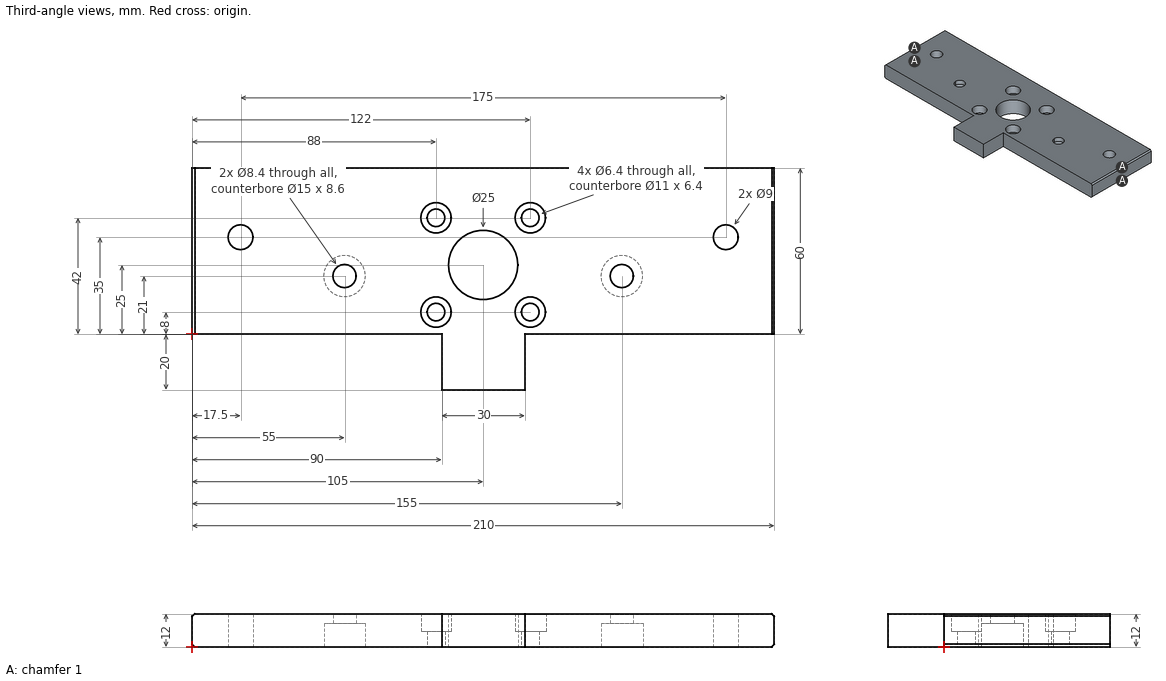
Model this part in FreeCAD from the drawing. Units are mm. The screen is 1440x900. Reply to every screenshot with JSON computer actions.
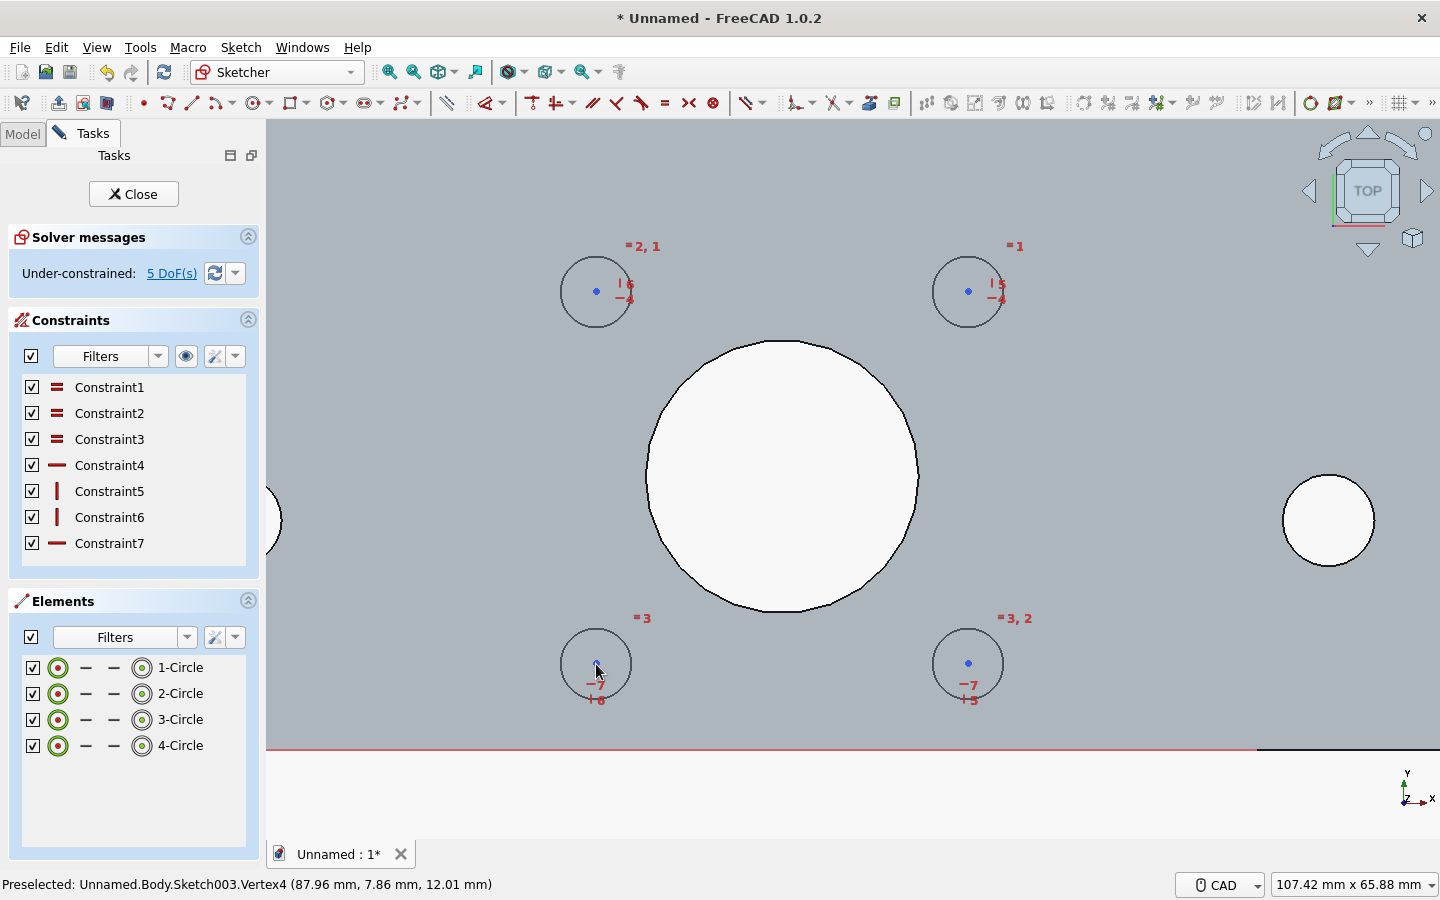
{"action": "key", "text": "d"}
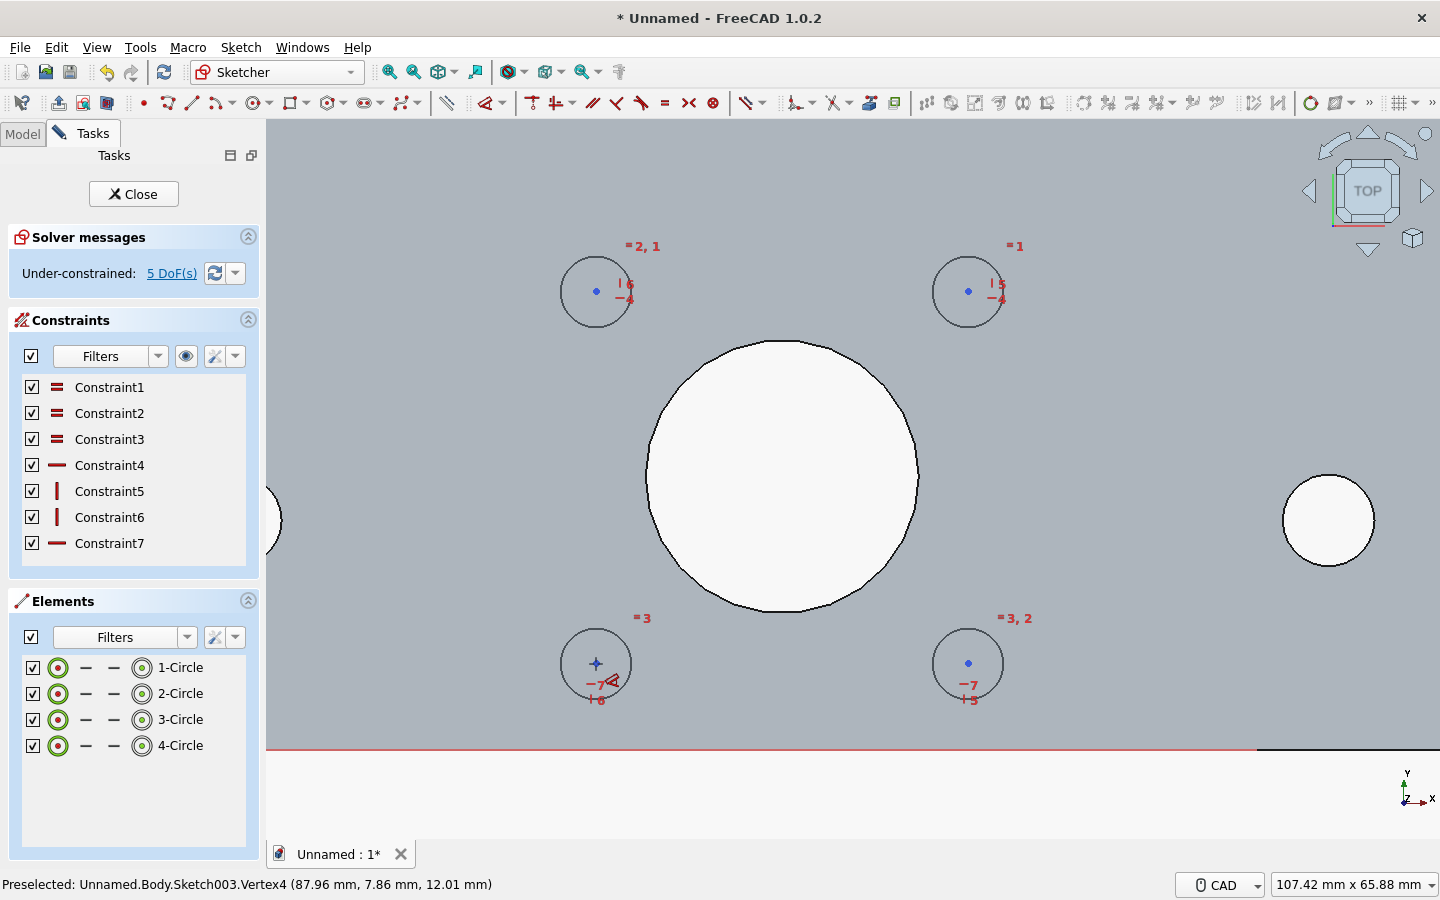
{"action": "left_click", "coordinate": [993, 267]}
{"action": "left_click", "coordinate": [1016, 244]}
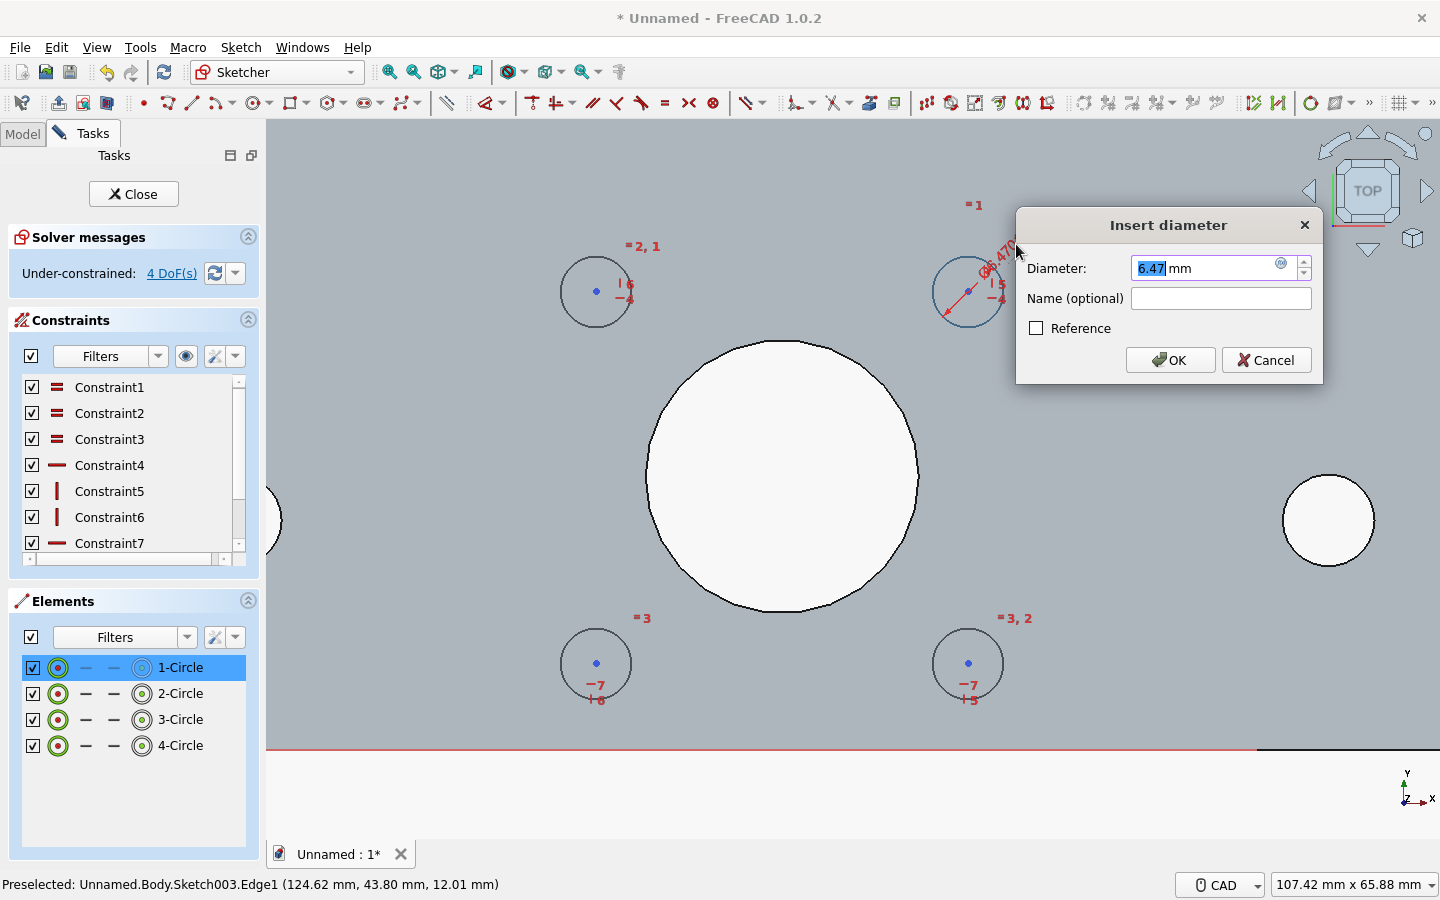
{"action": "type", "text": "6.4"}
{"action": "key", "text": "Return"}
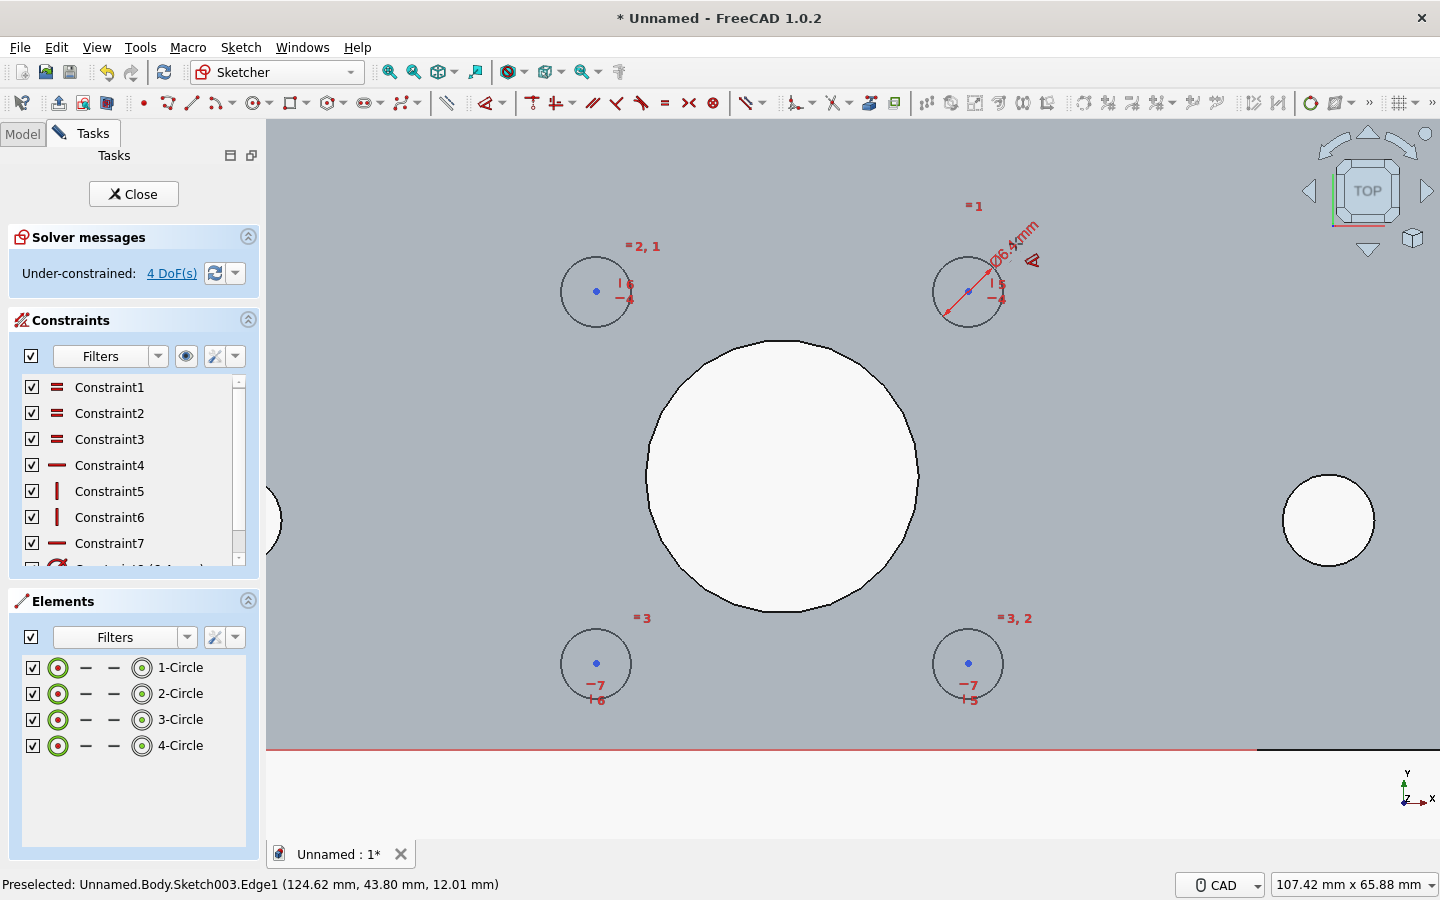
{"action": "left_click", "coordinate": [968, 664]}
{"action": "left_click", "coordinate": [1002, 707]}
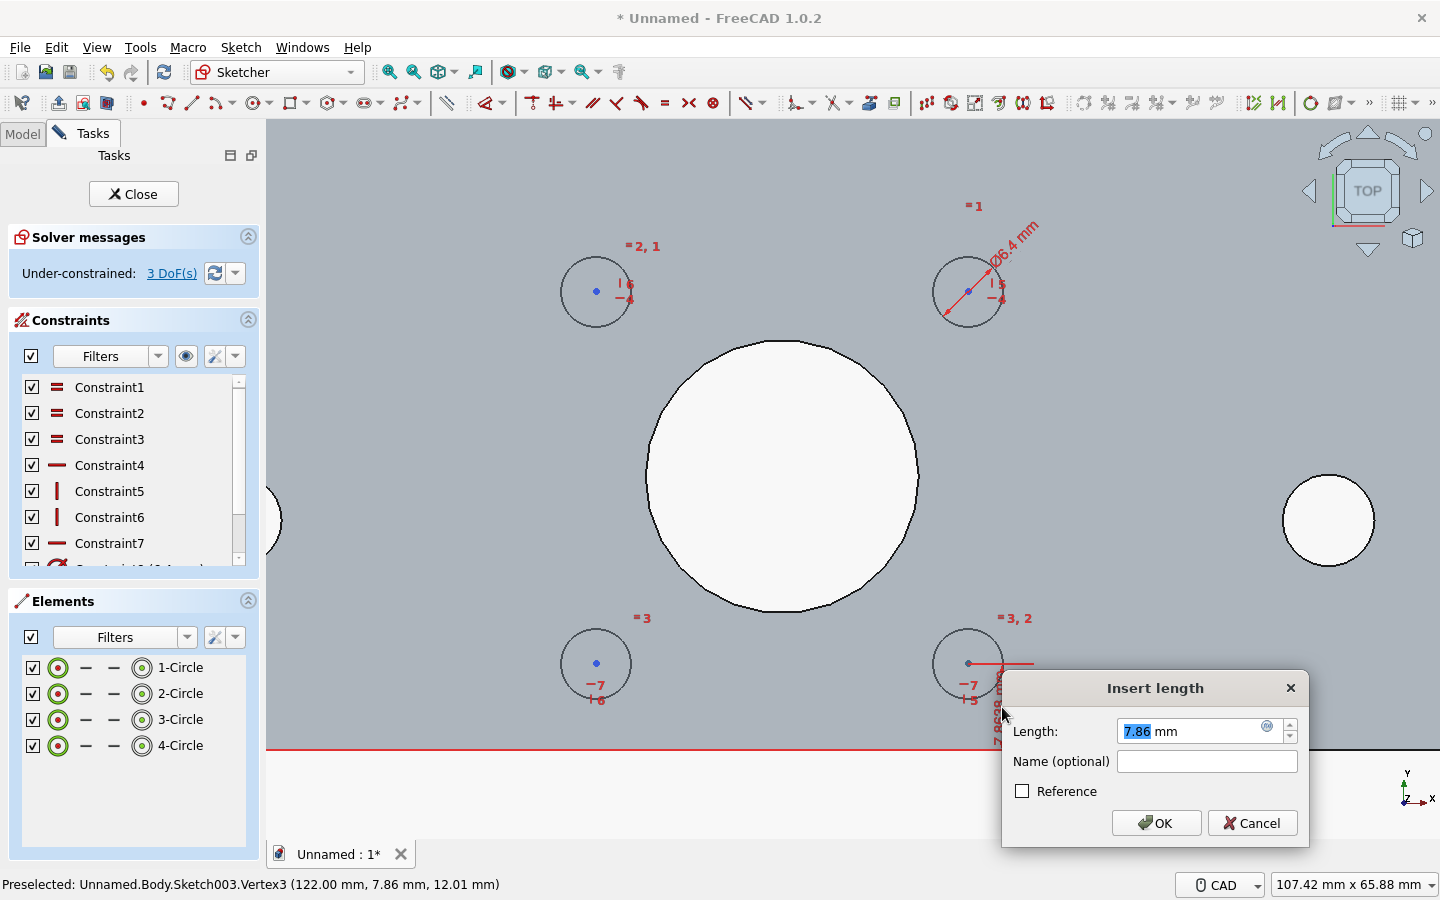
{"action": "type", "text": "8"}
{"action": "key", "text": "Return"}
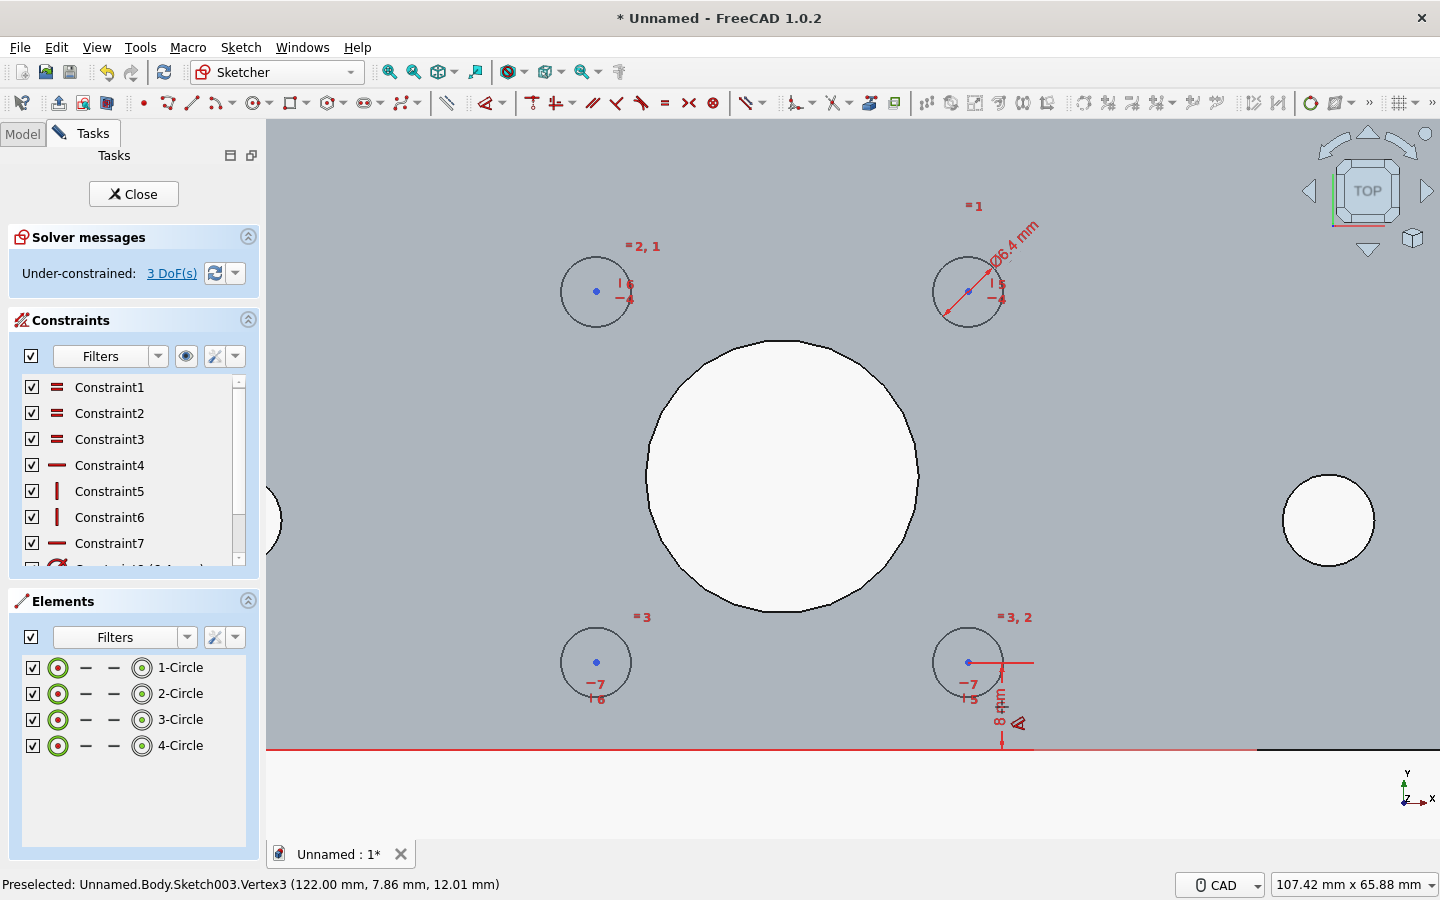
{"action": "left_click", "coordinate": [968, 292]}
{"action": "left_click", "coordinate": [1002, 521]}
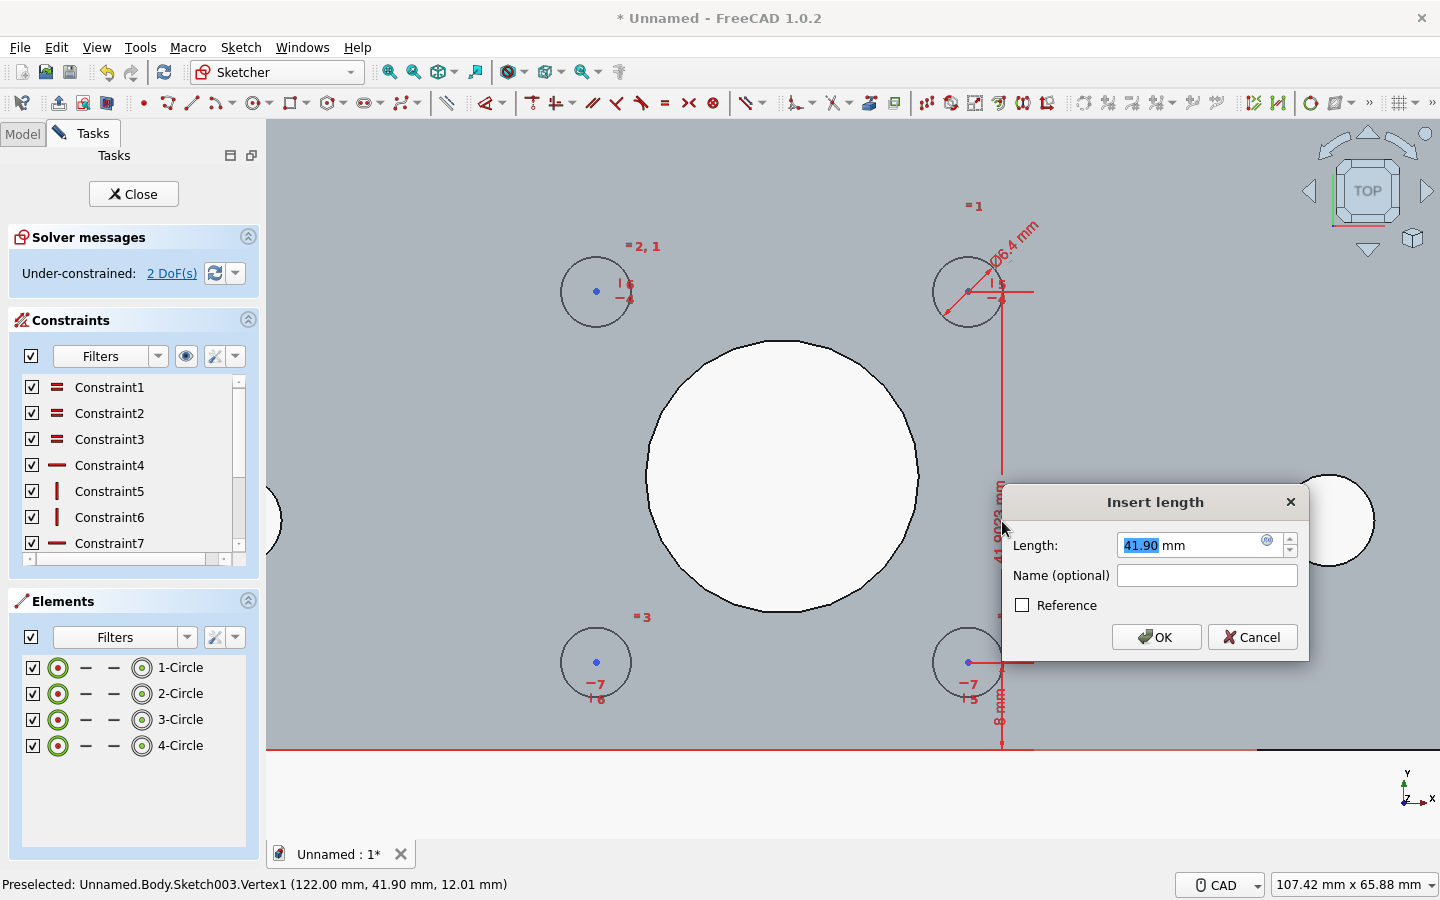
{"action": "type", "text": "42"}
{"action": "key", "text": "Return"}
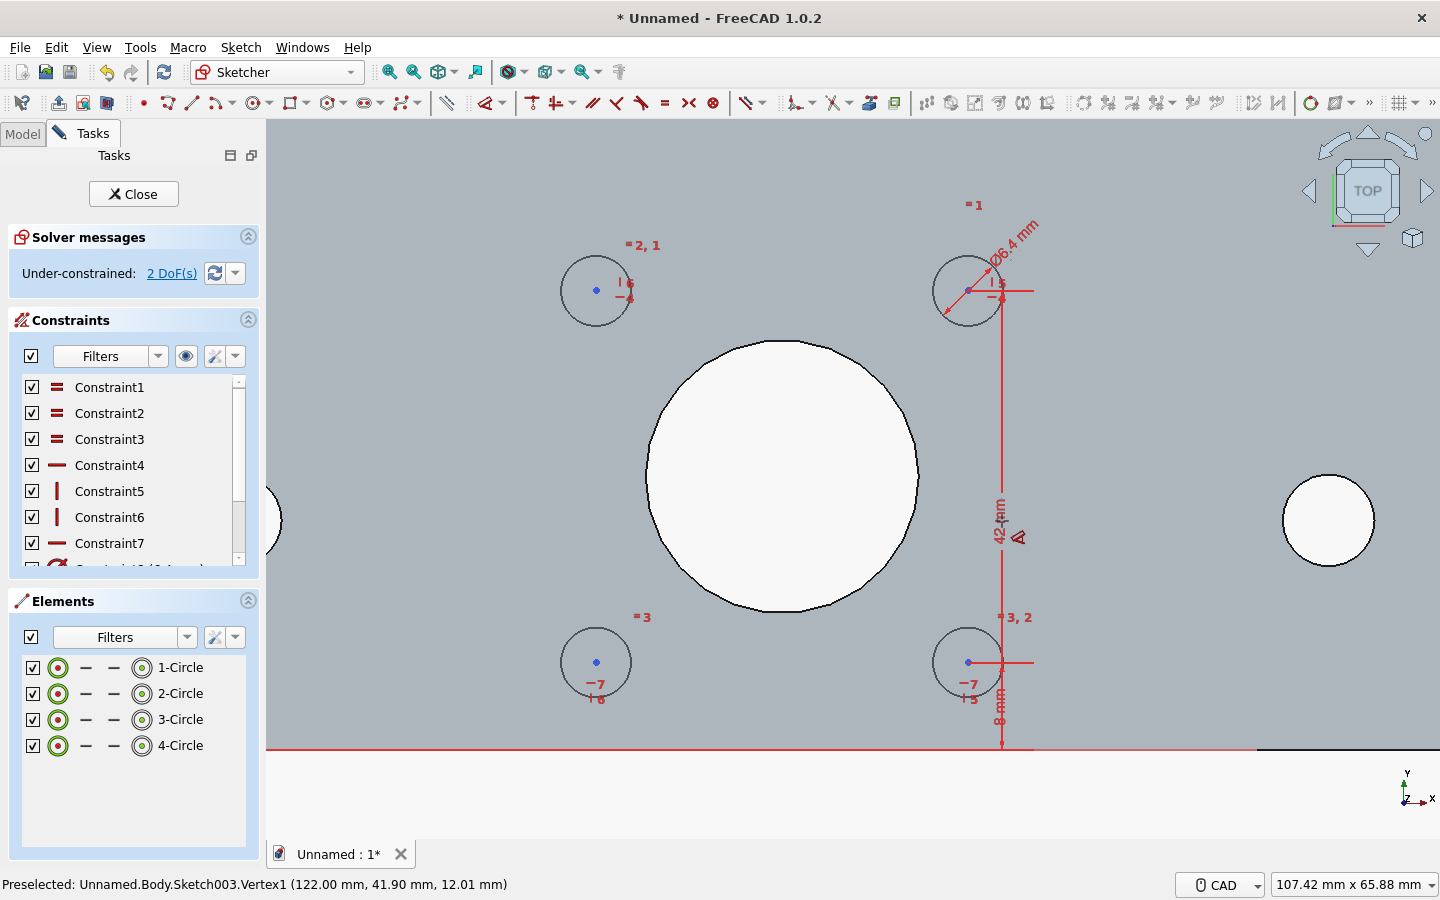
{"action": "left_click", "coordinate": [596, 291]}
{"action": "left_click", "coordinate": [445, 784]}